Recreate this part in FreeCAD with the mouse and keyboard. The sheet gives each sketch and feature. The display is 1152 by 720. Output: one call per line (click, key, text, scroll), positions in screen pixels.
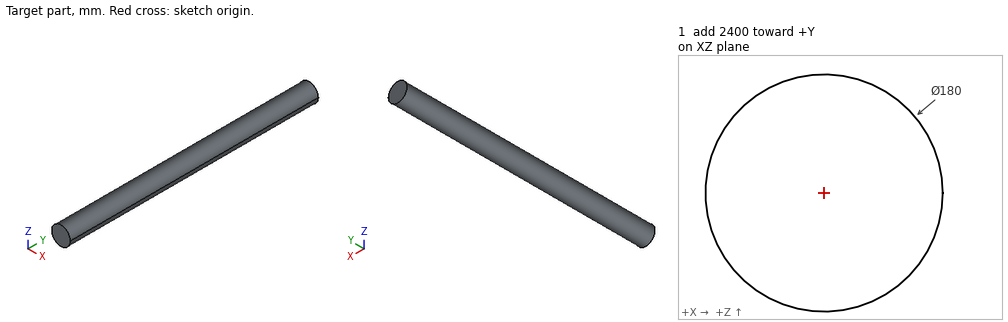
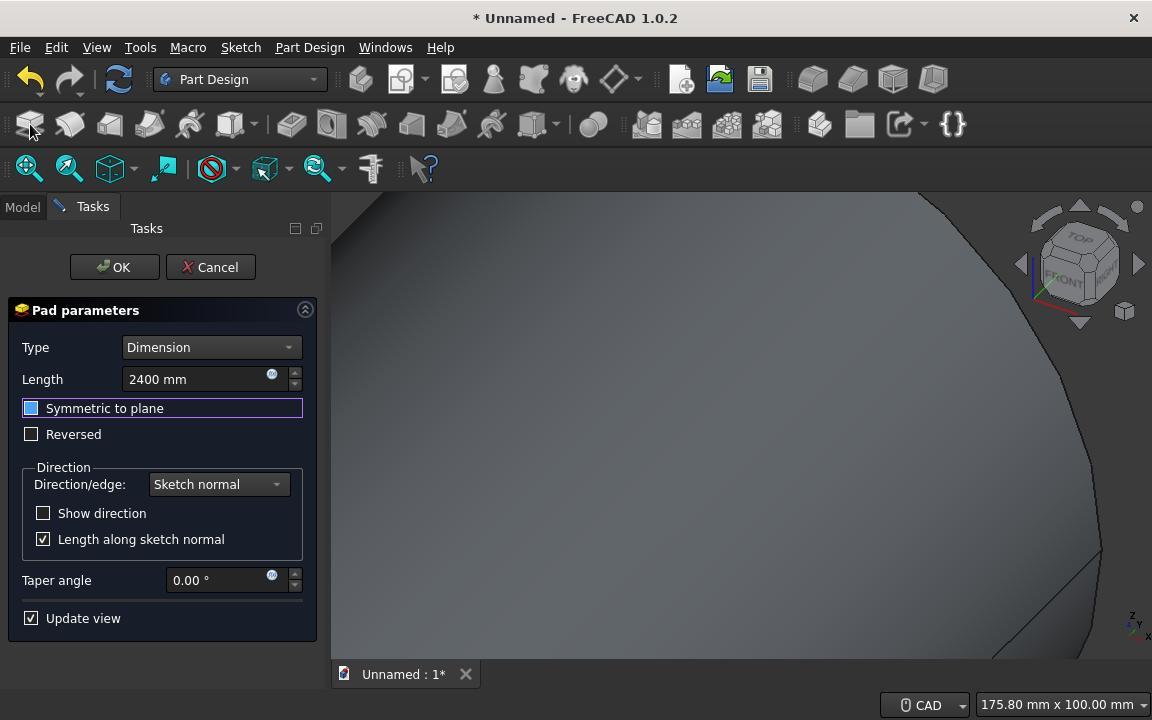
click(30, 434)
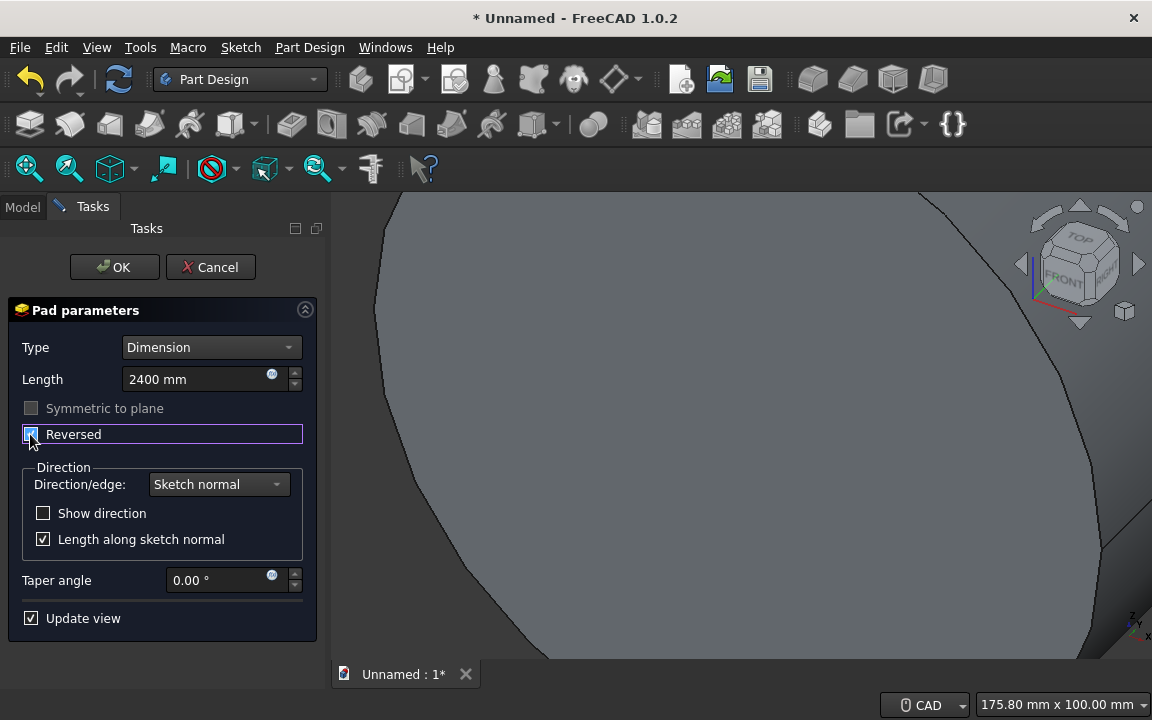
click(115, 267)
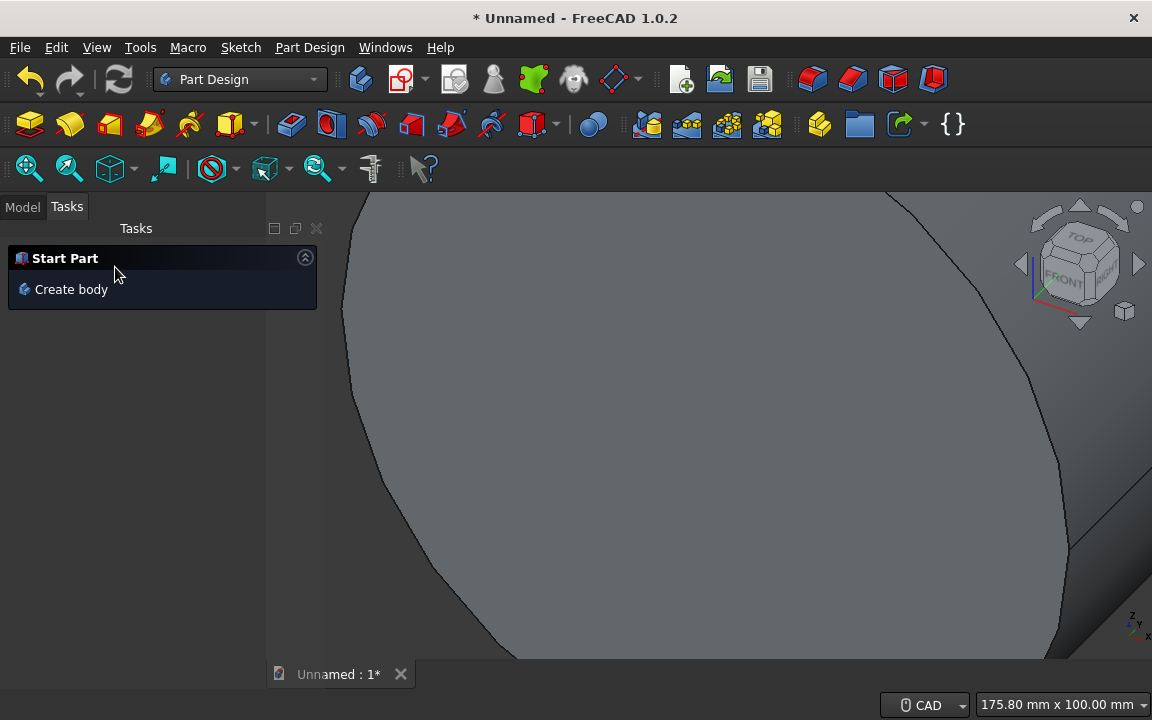
key(0)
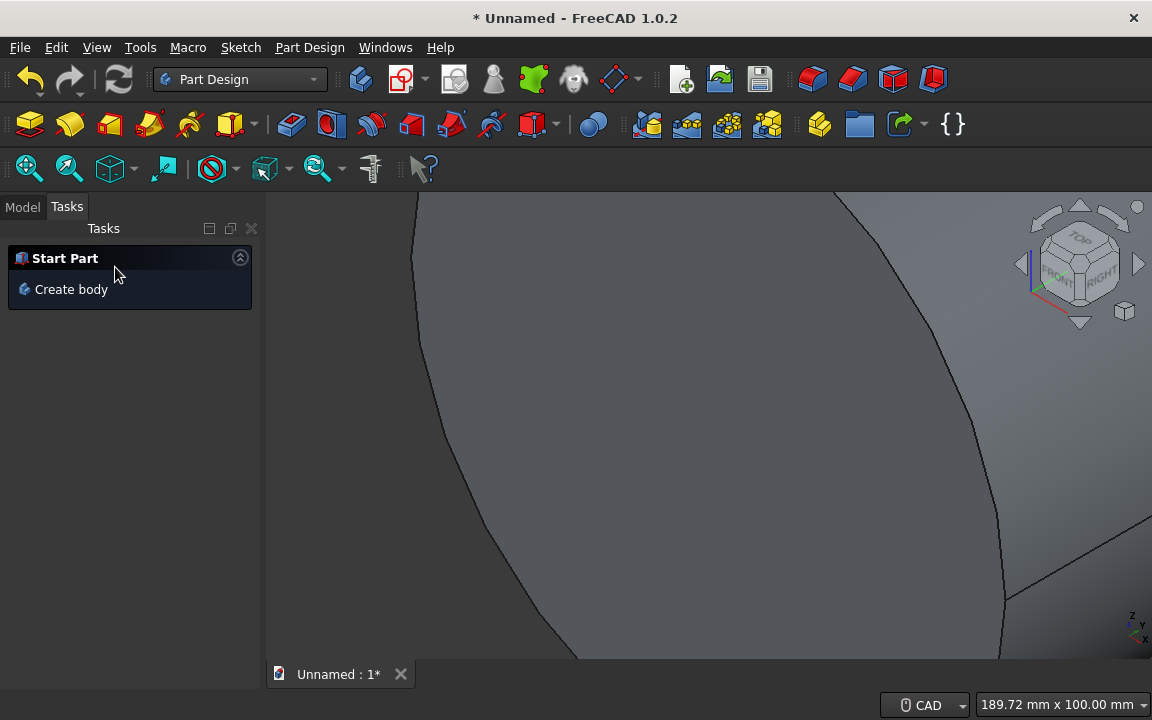
key(v)
key(f)